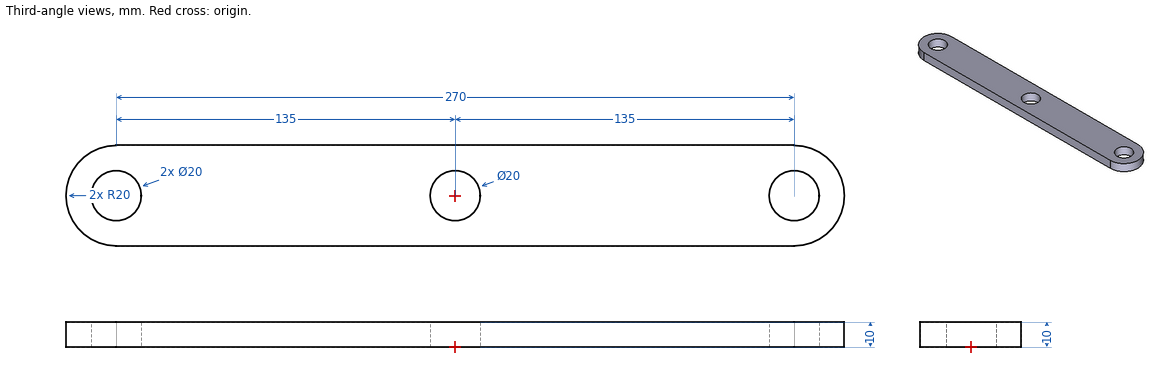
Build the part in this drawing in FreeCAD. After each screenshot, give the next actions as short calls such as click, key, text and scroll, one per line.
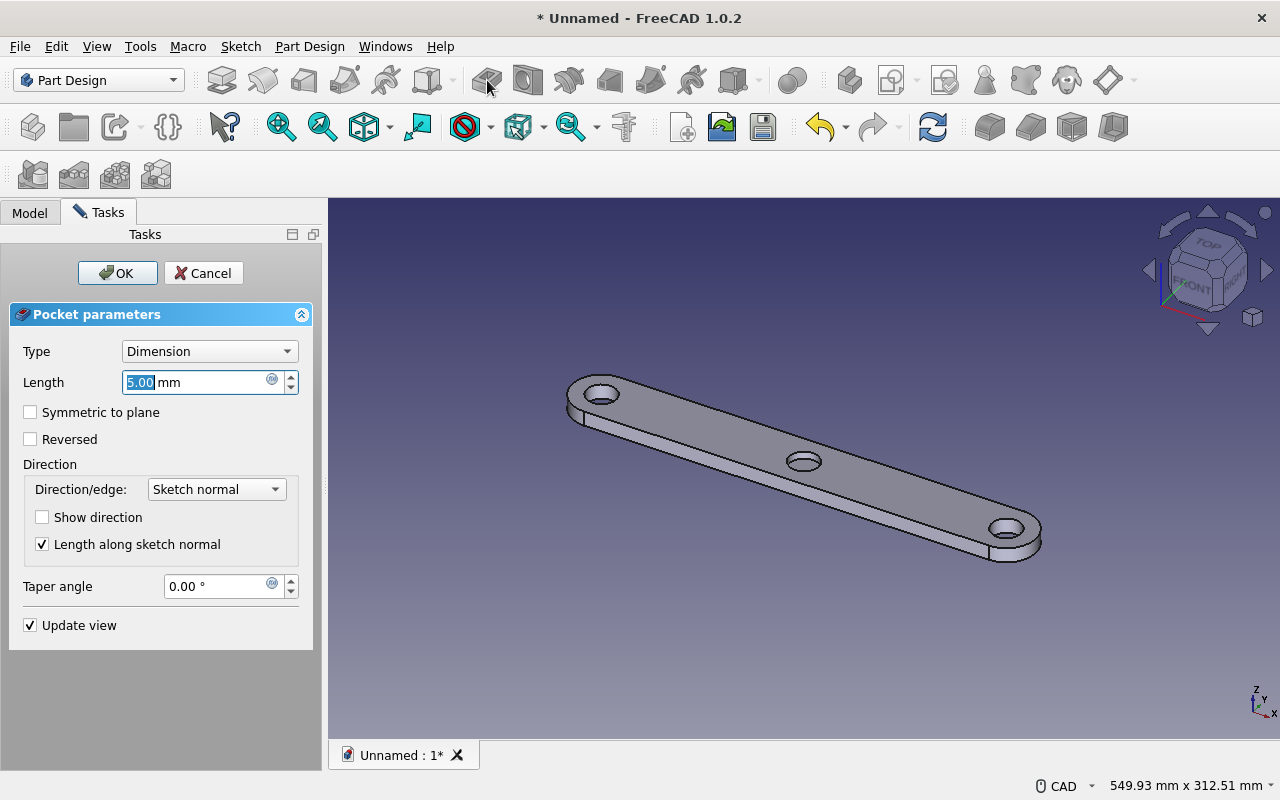
text(10)
key(Tab)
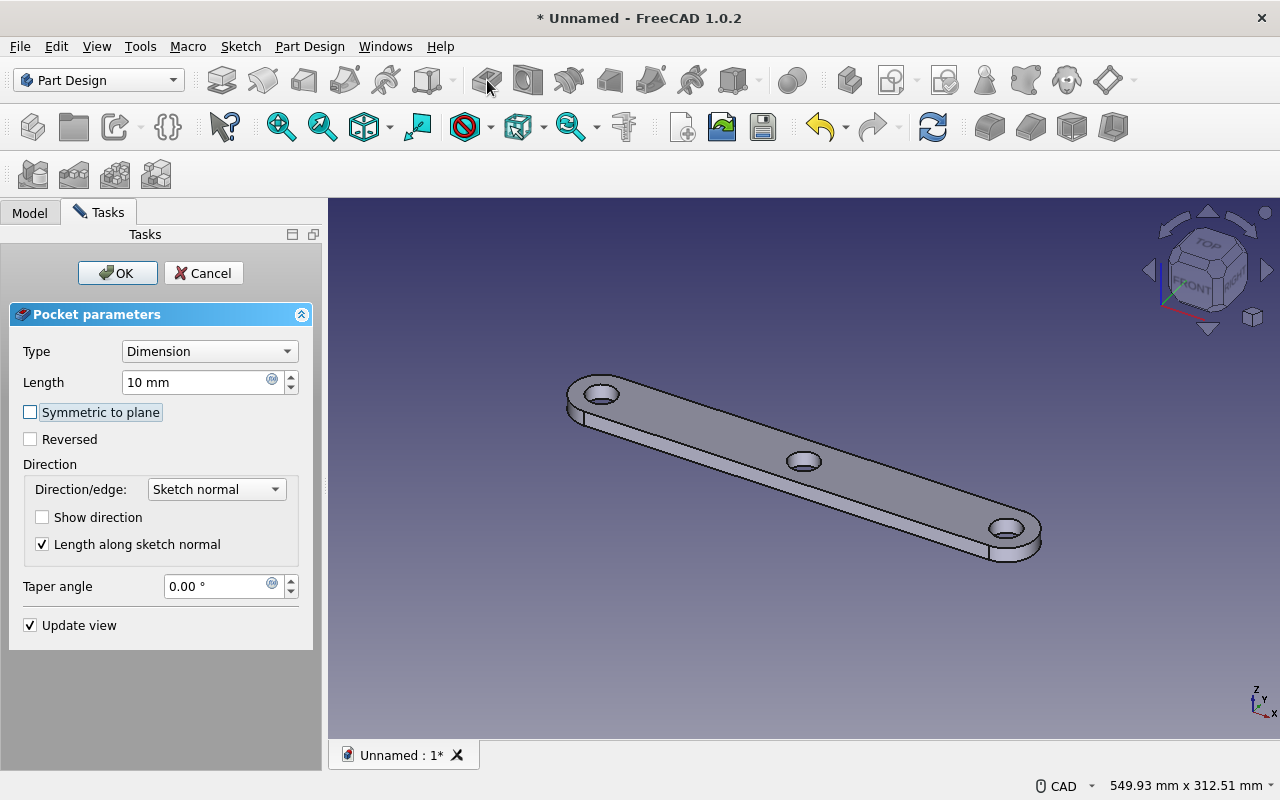
click(118, 273)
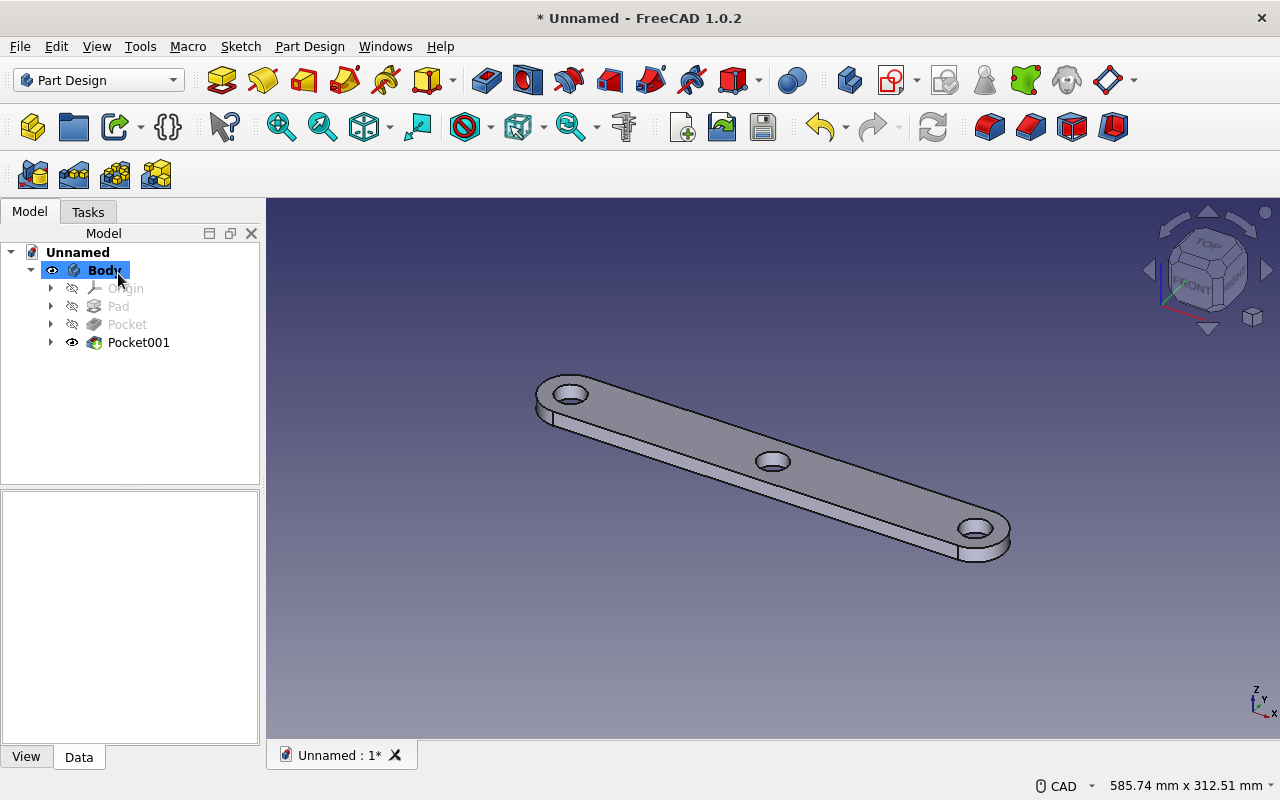
key(0)